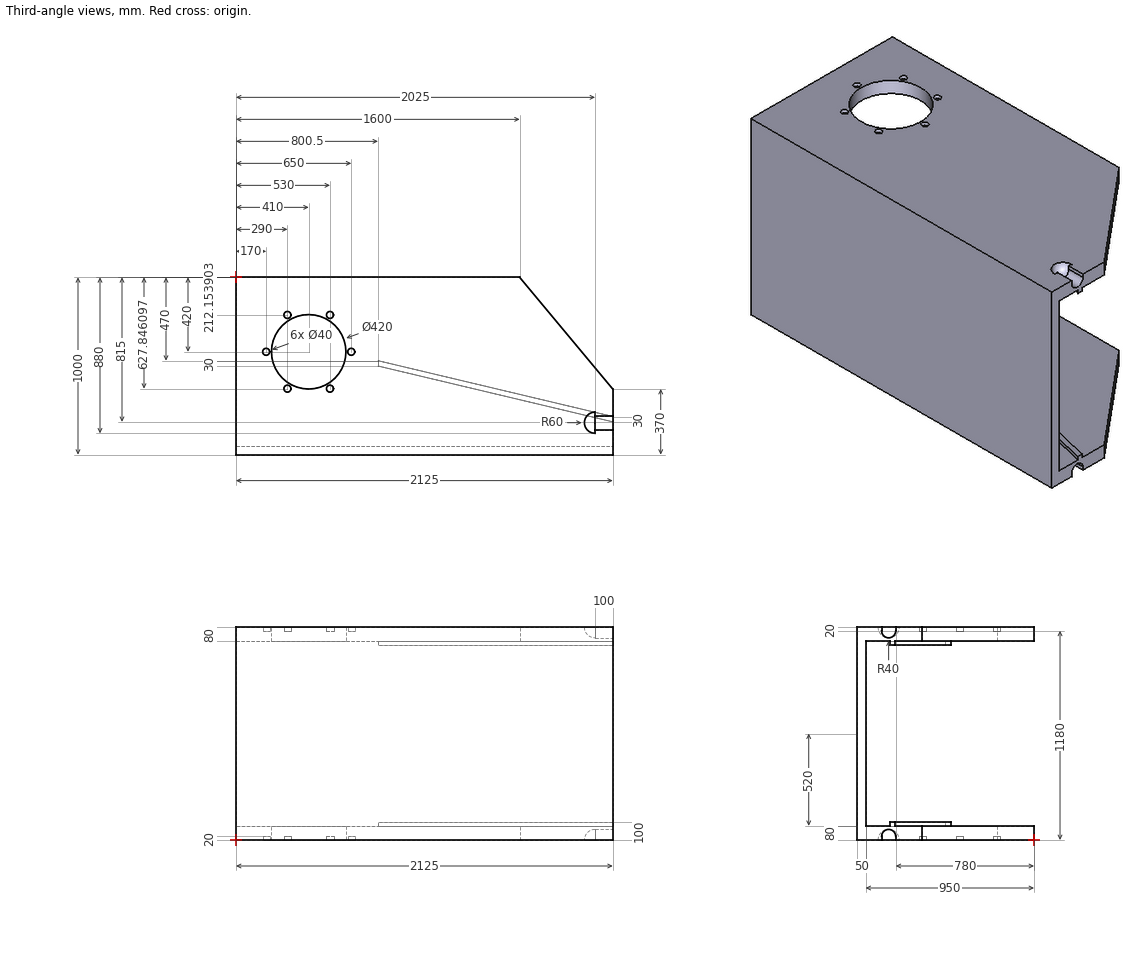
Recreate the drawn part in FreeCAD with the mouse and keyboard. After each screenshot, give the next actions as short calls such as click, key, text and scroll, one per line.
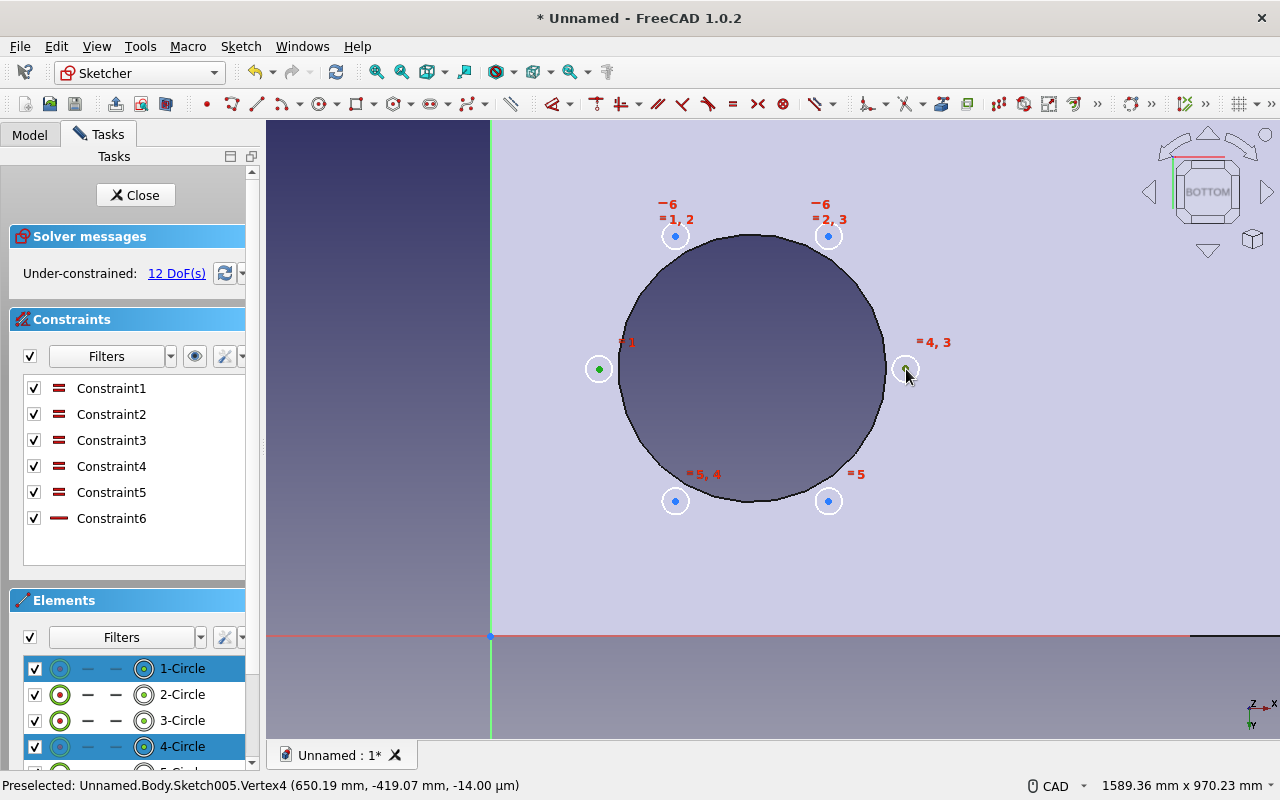
key(h)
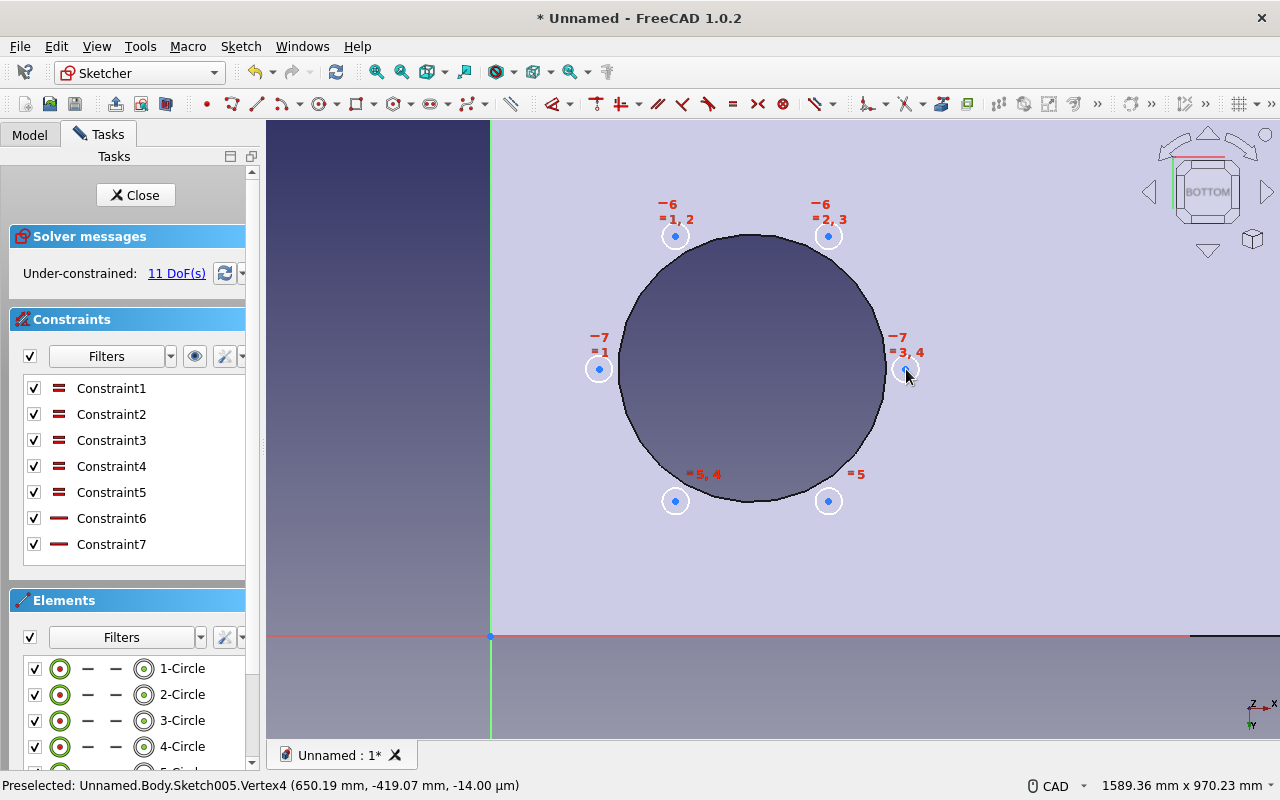
click(676, 236)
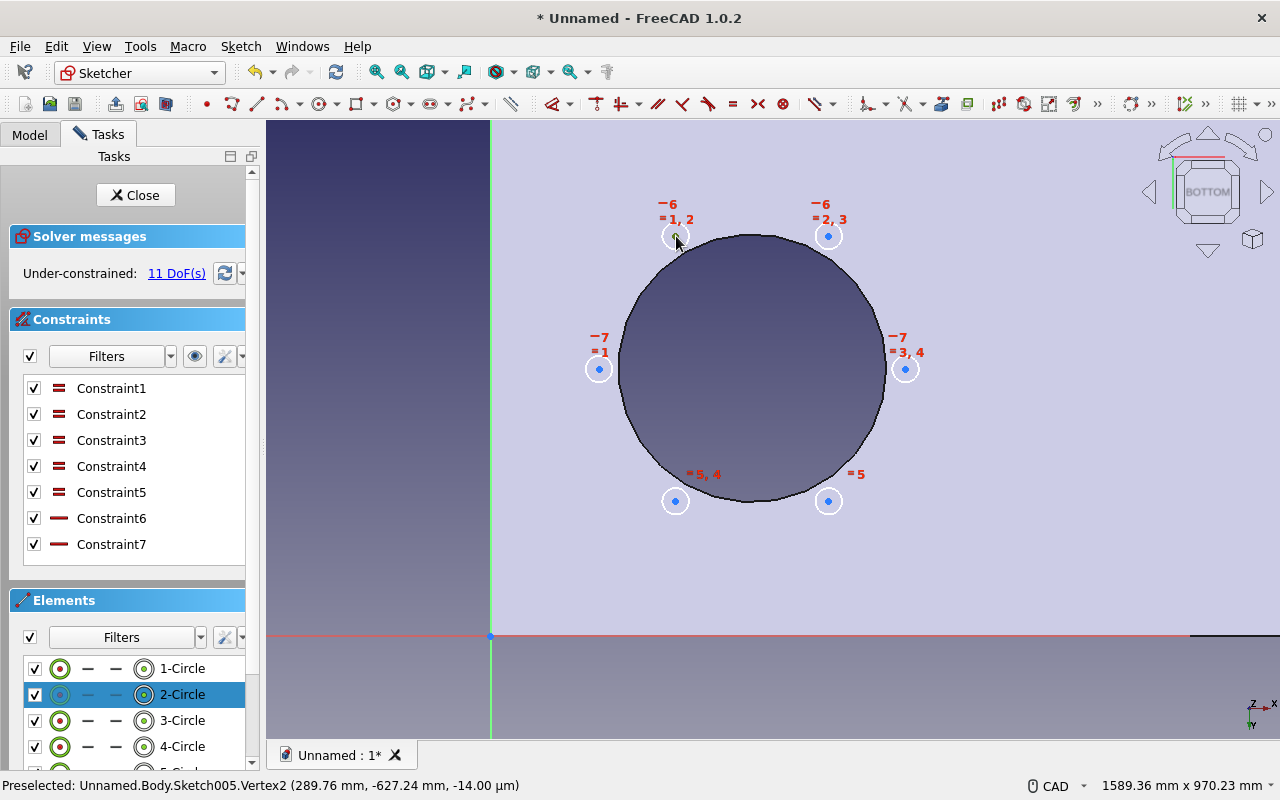
click(676, 501)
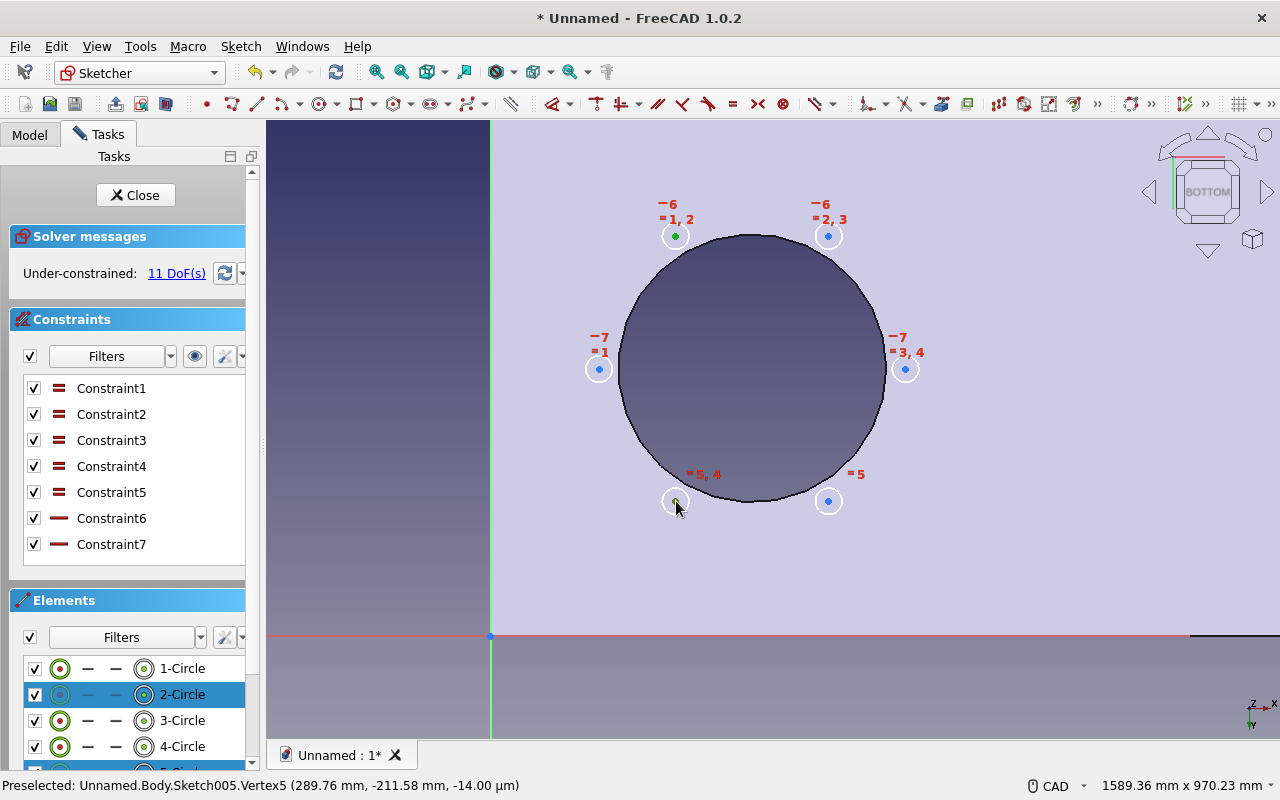
click(638, 104)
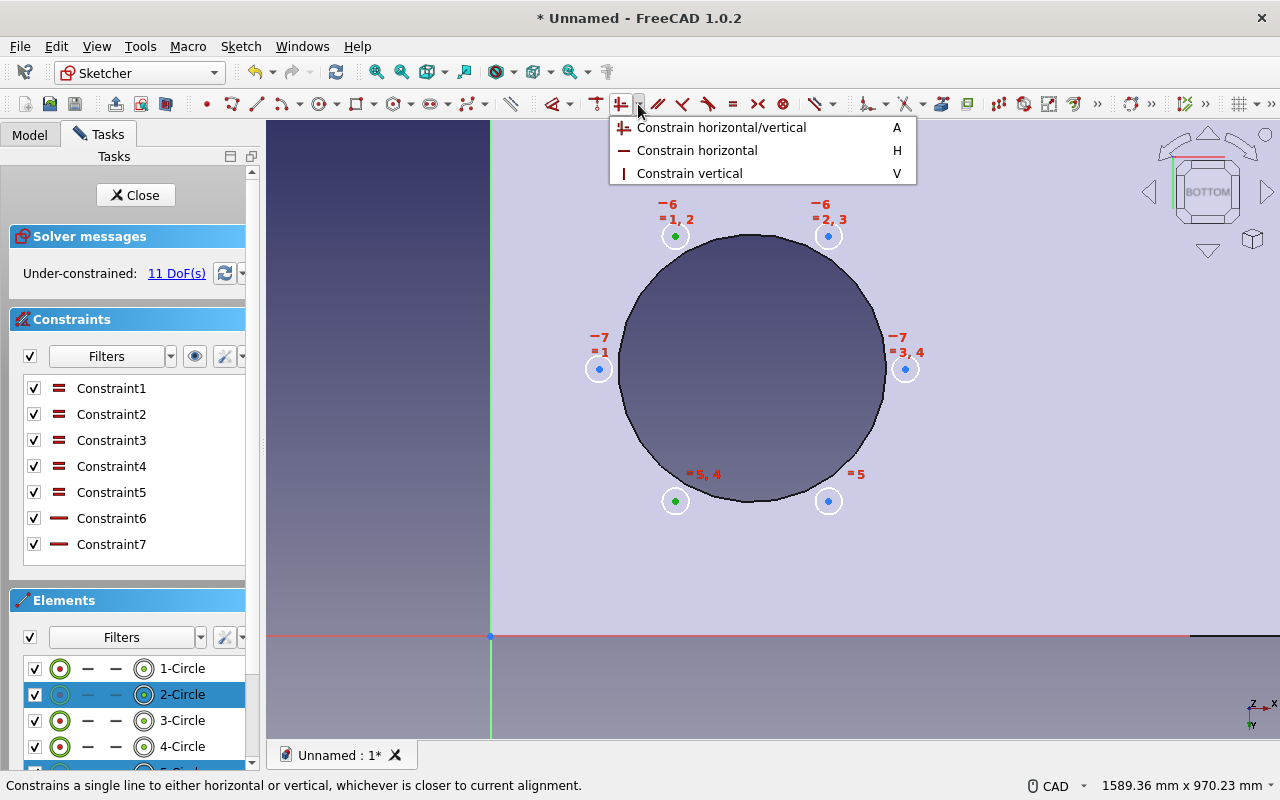
click(763, 174)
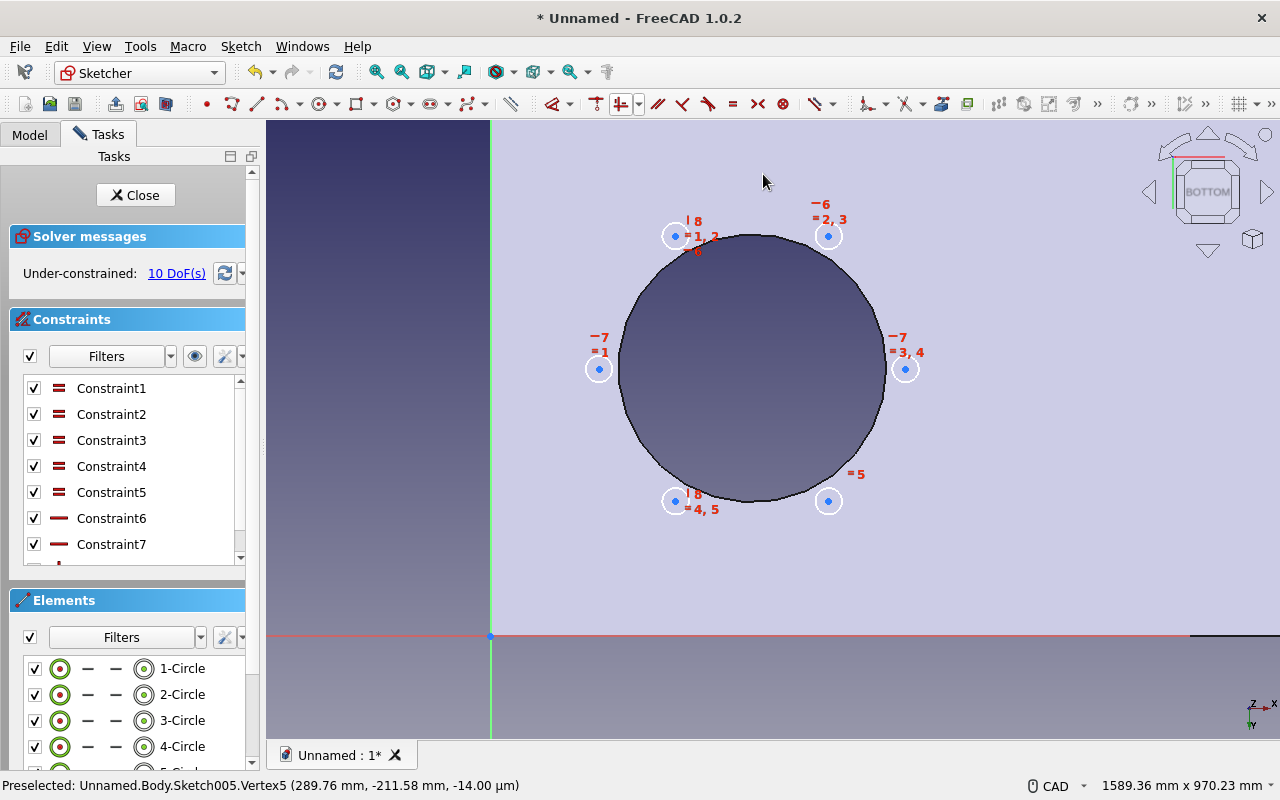
click(829, 236)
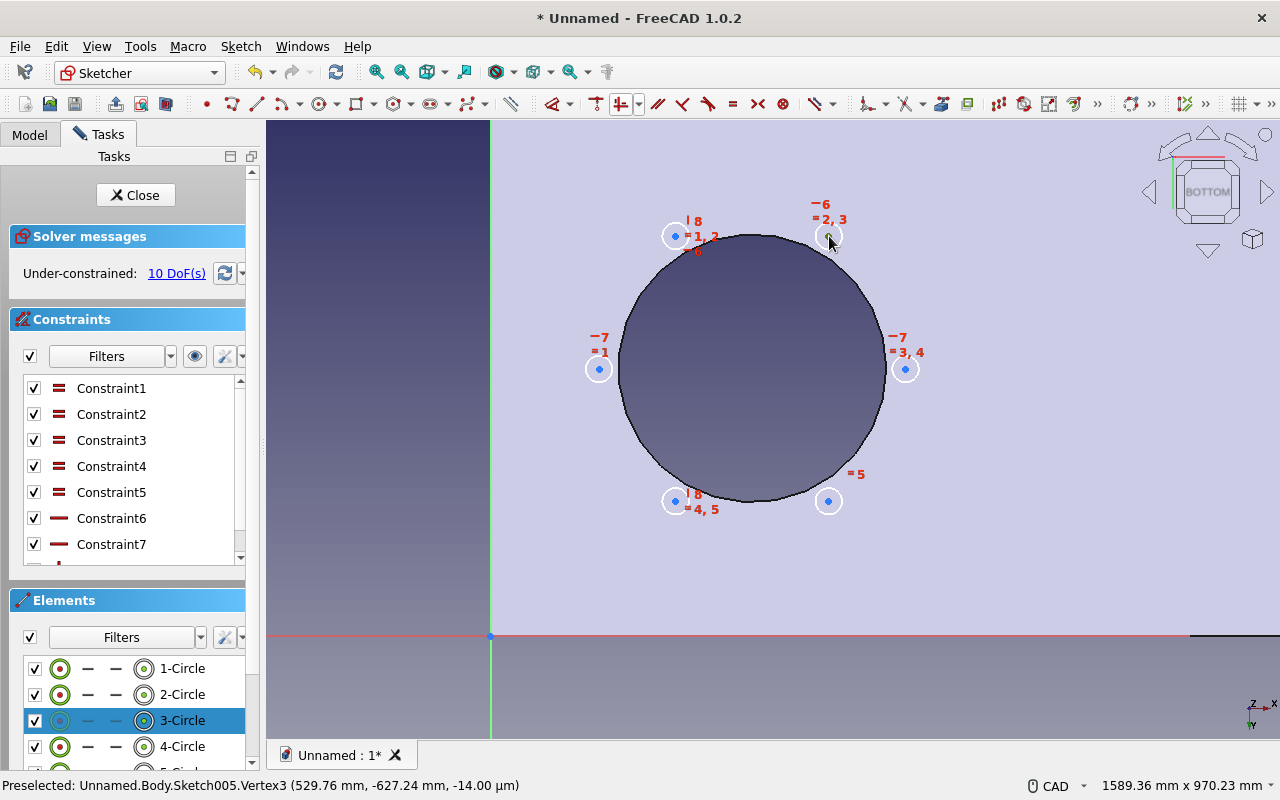
click(829, 501)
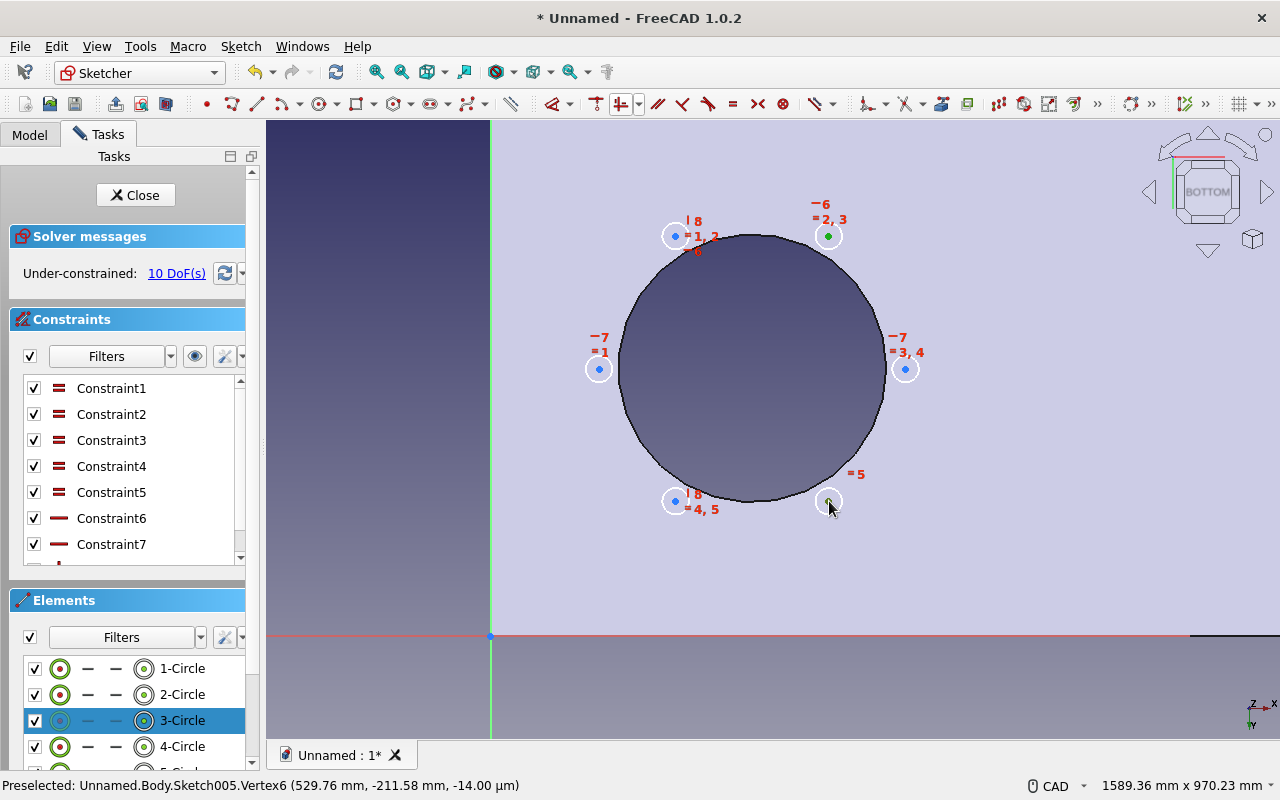
key(v)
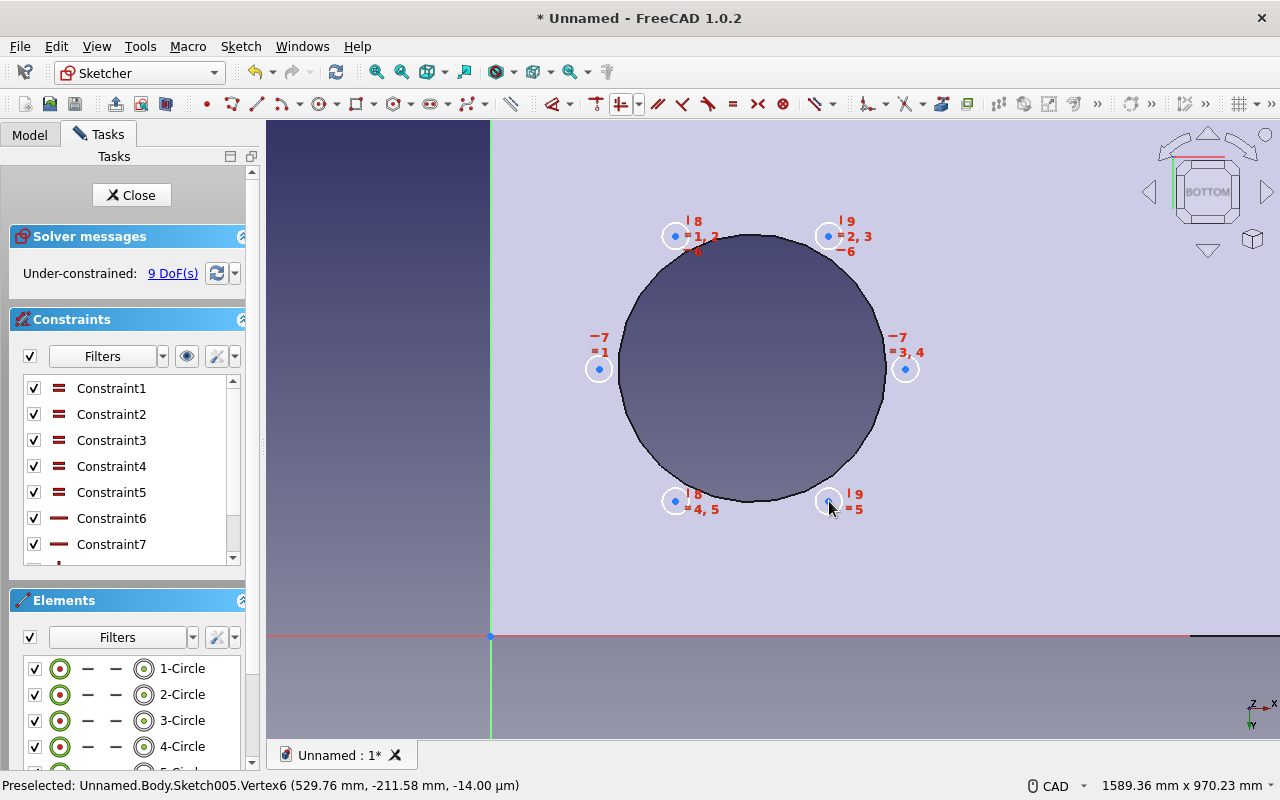
click(676, 501)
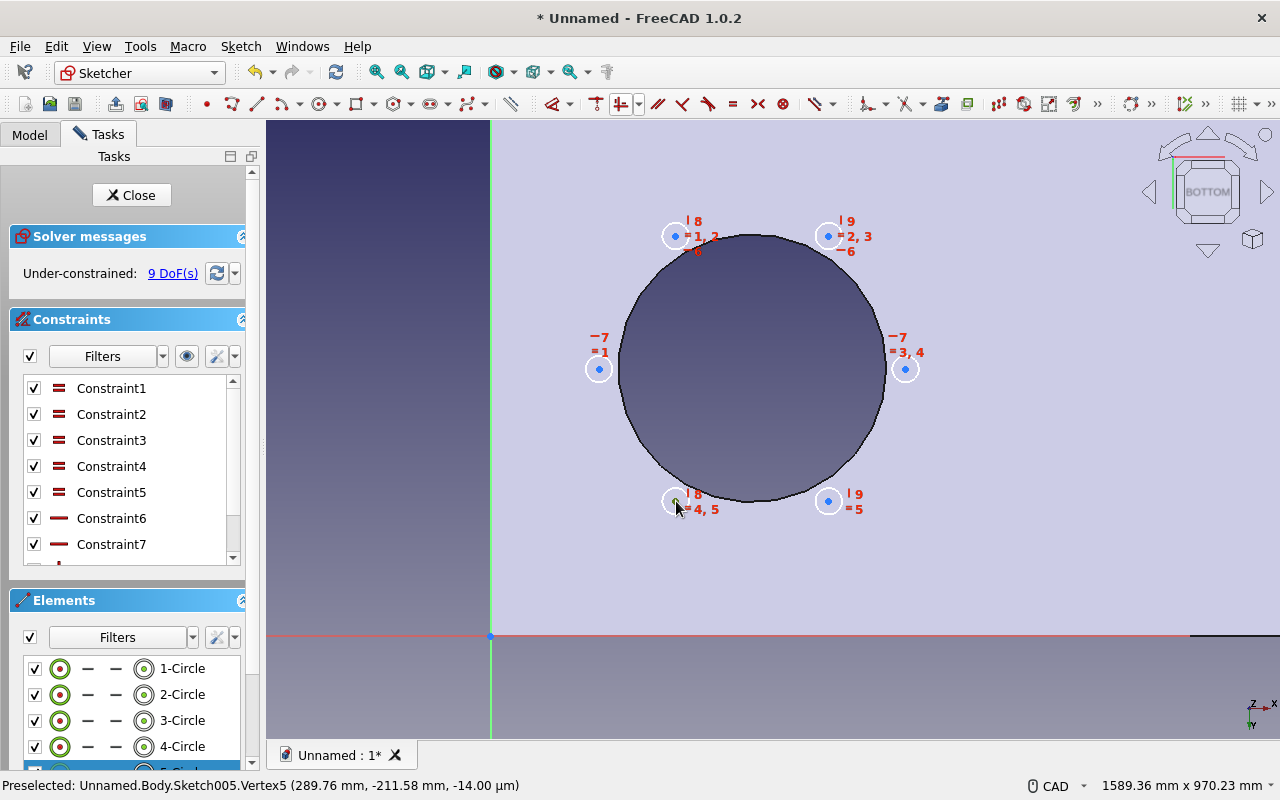
click(829, 501)